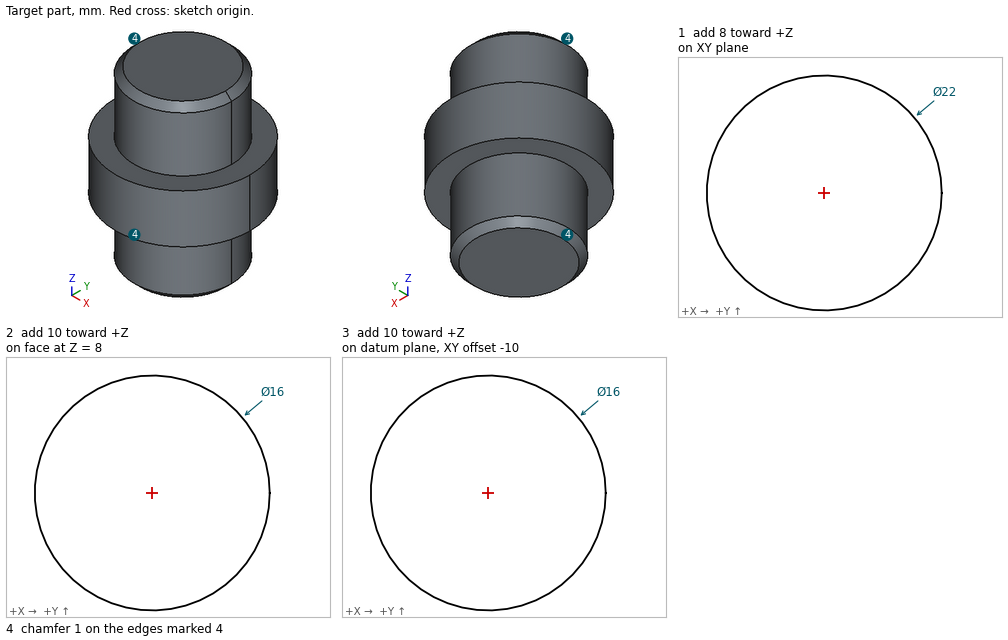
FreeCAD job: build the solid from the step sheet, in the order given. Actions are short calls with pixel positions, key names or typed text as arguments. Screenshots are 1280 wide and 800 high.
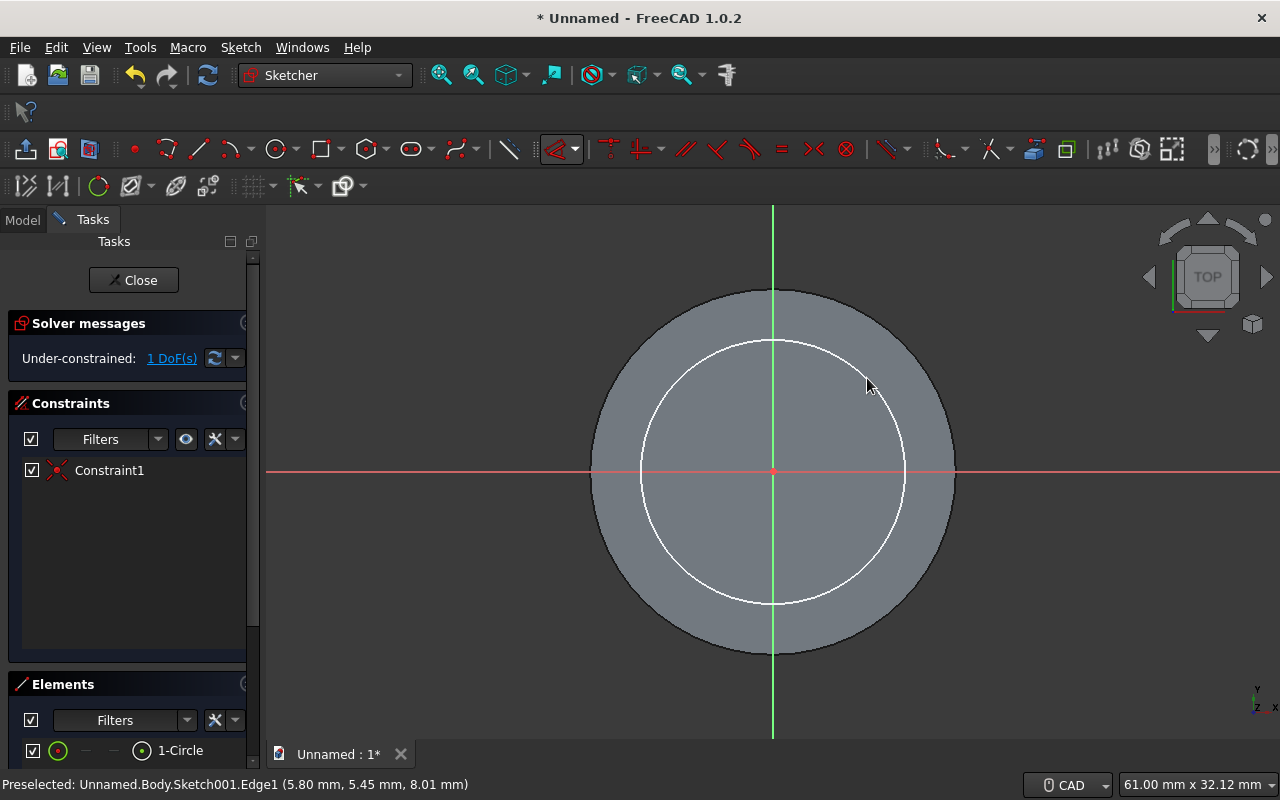
click(866, 378)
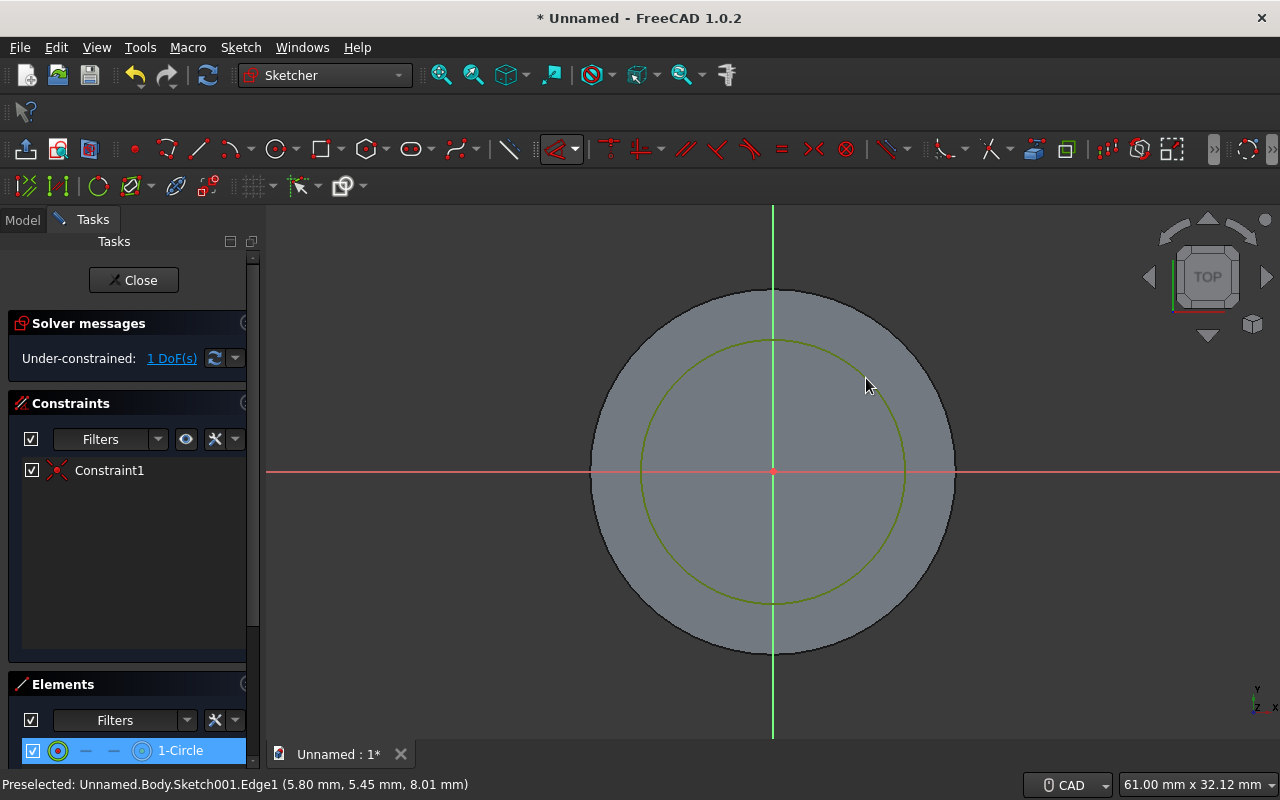
key(k)
key(o)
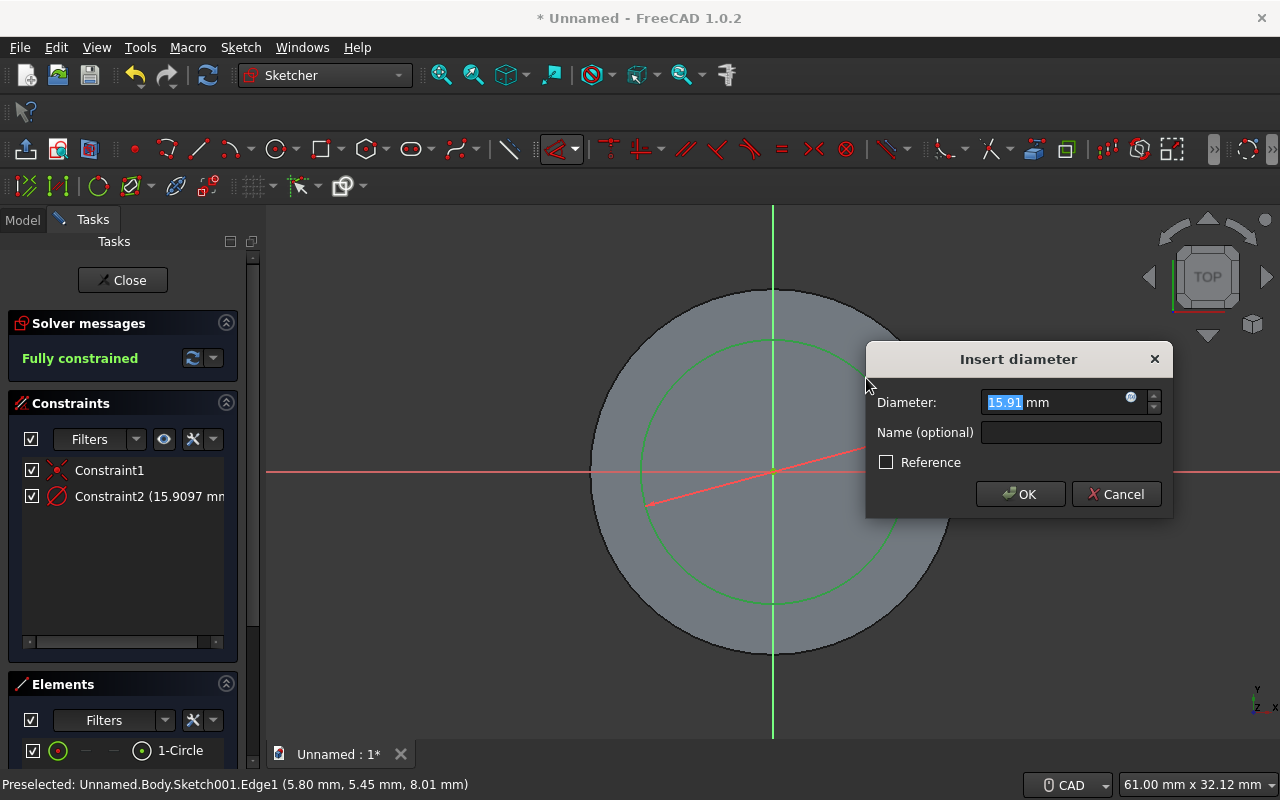
text(16)
key(Return)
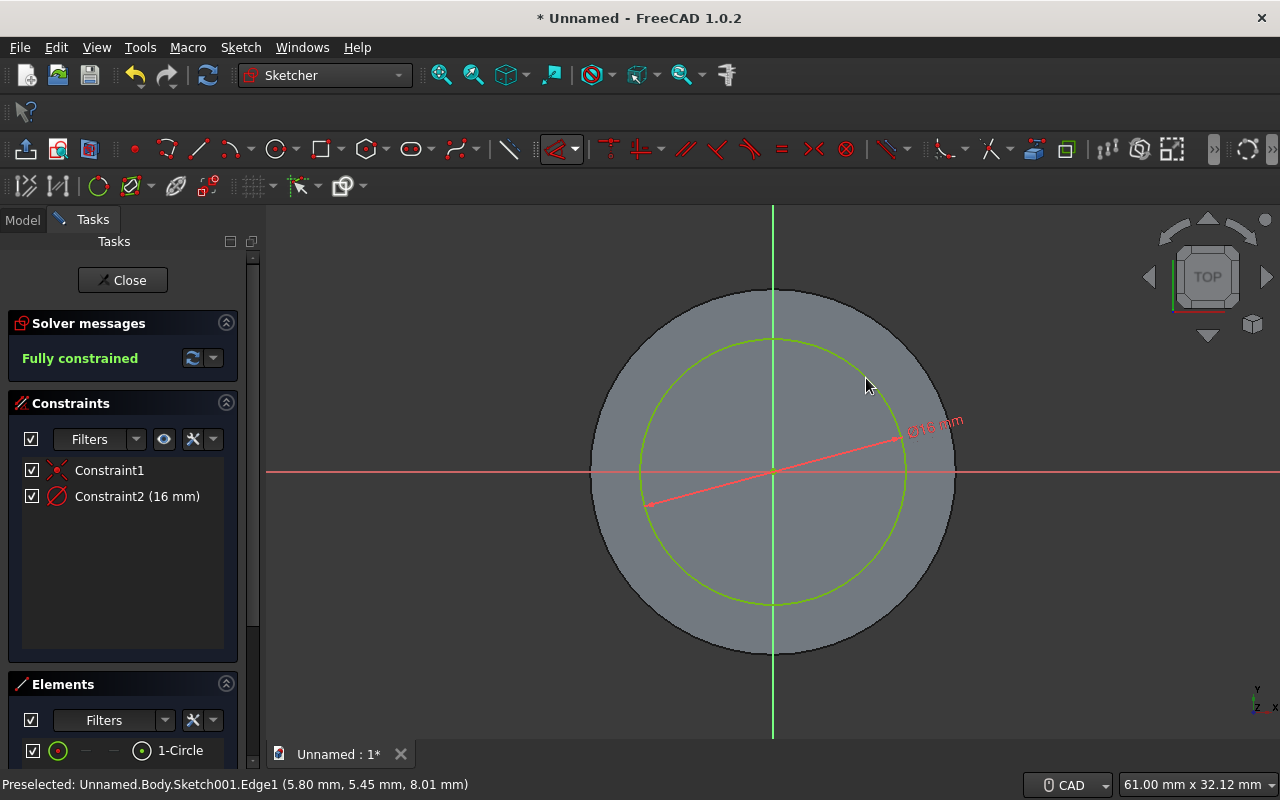
click(123, 280)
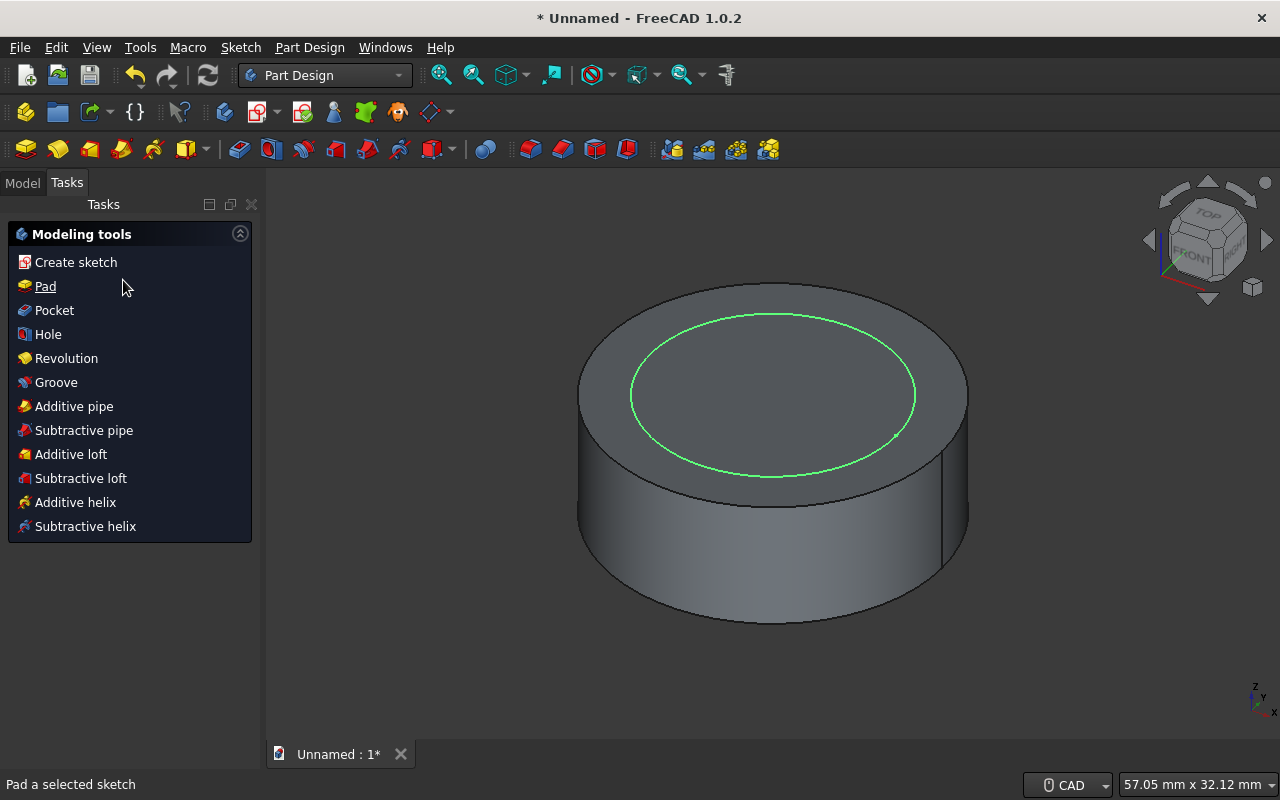
click(26, 150)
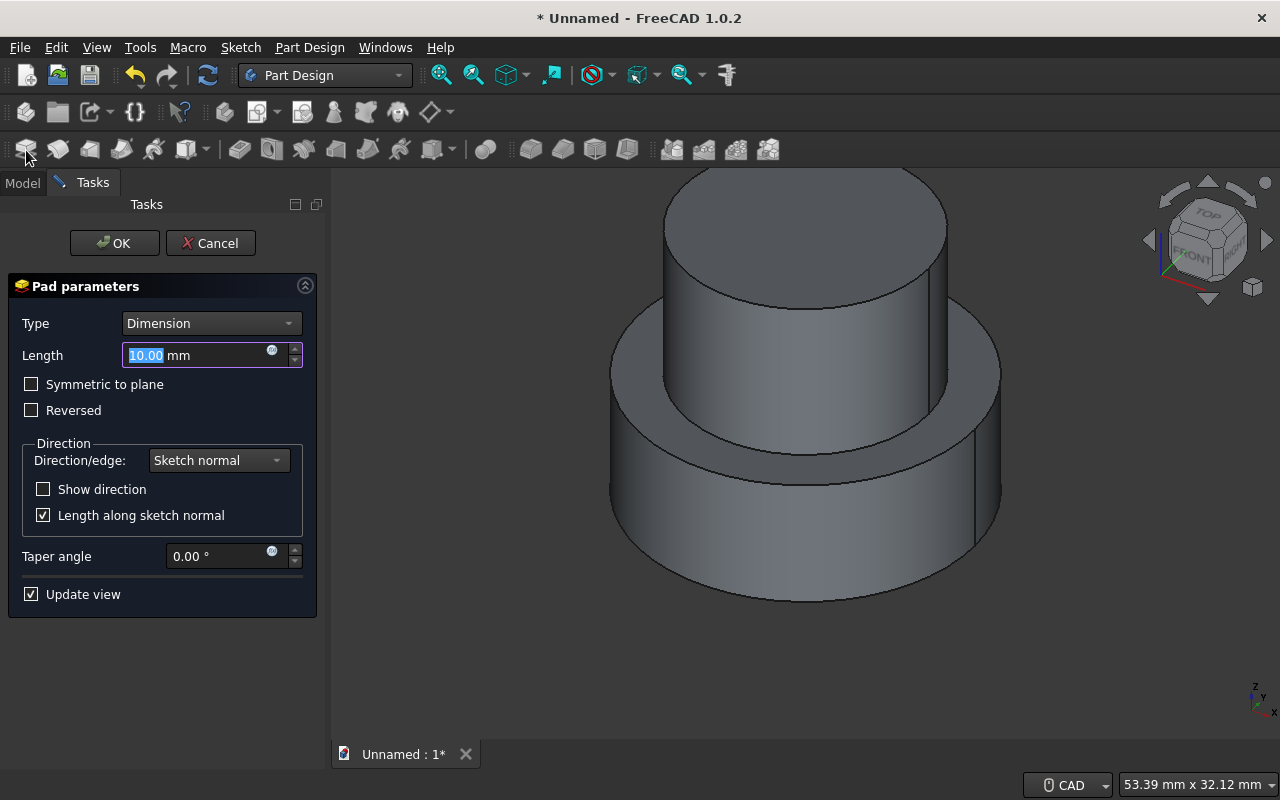
text(10)
key(Tab)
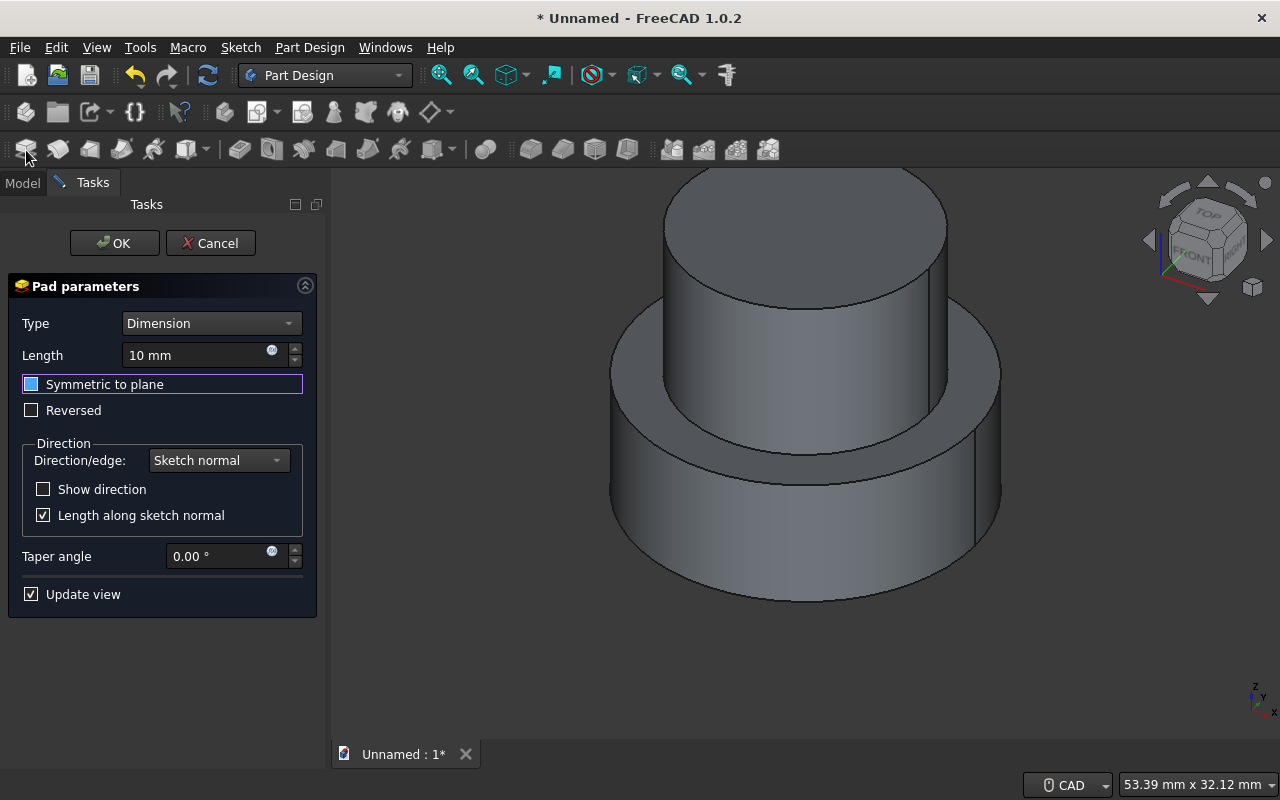
click(115, 243)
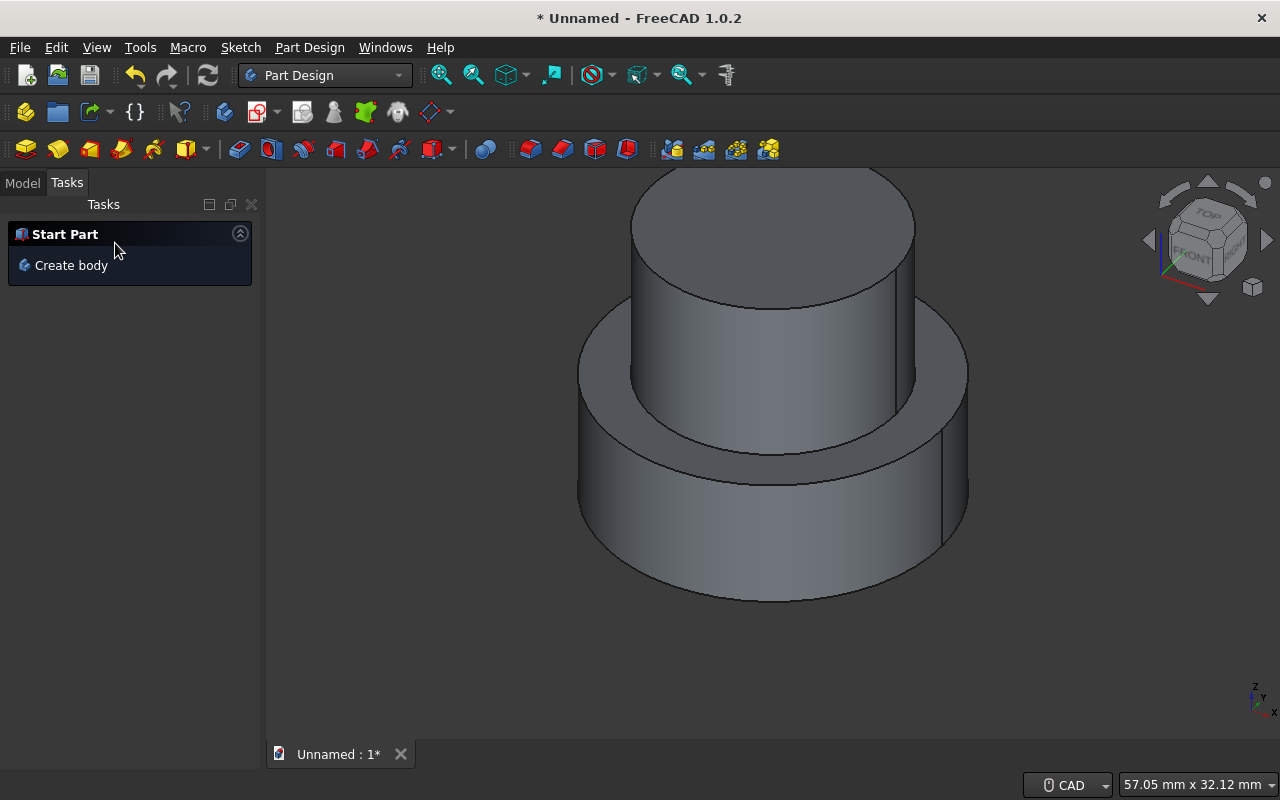
key(v)
key(f)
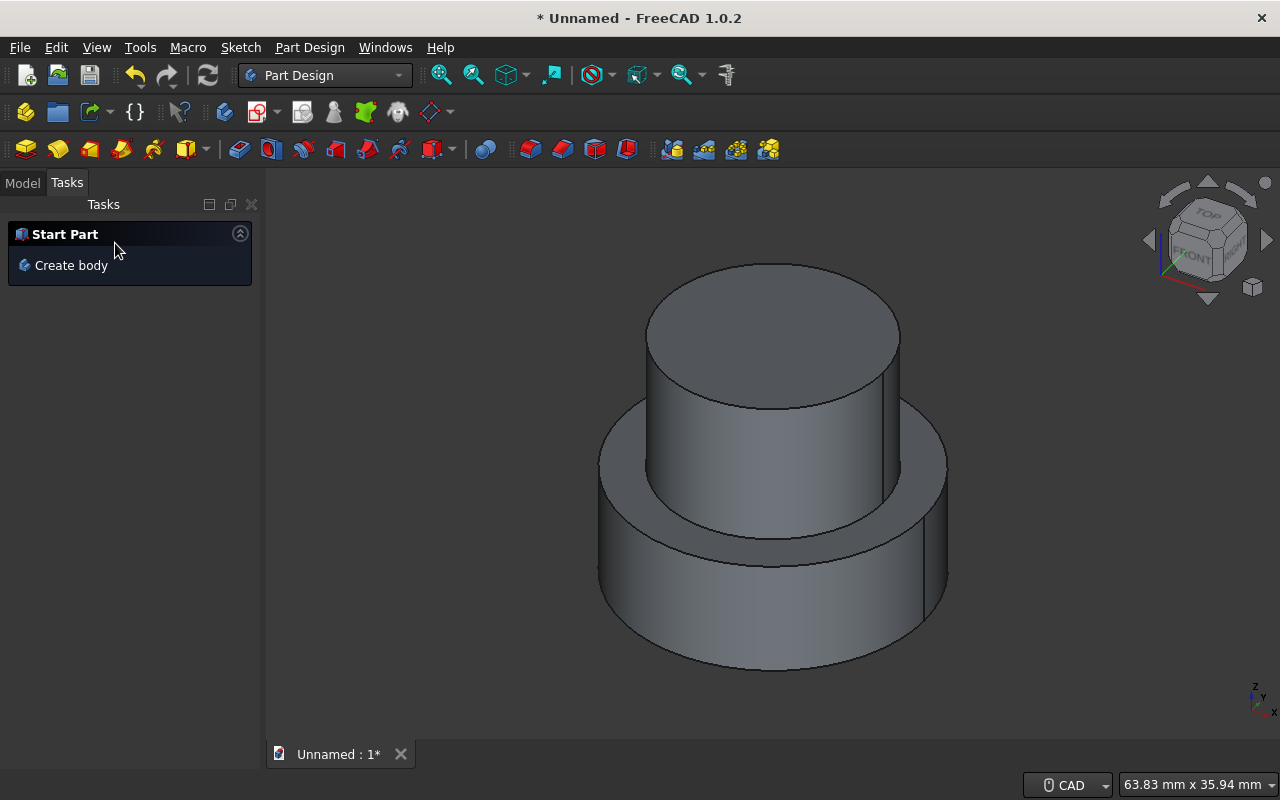
click(23, 182)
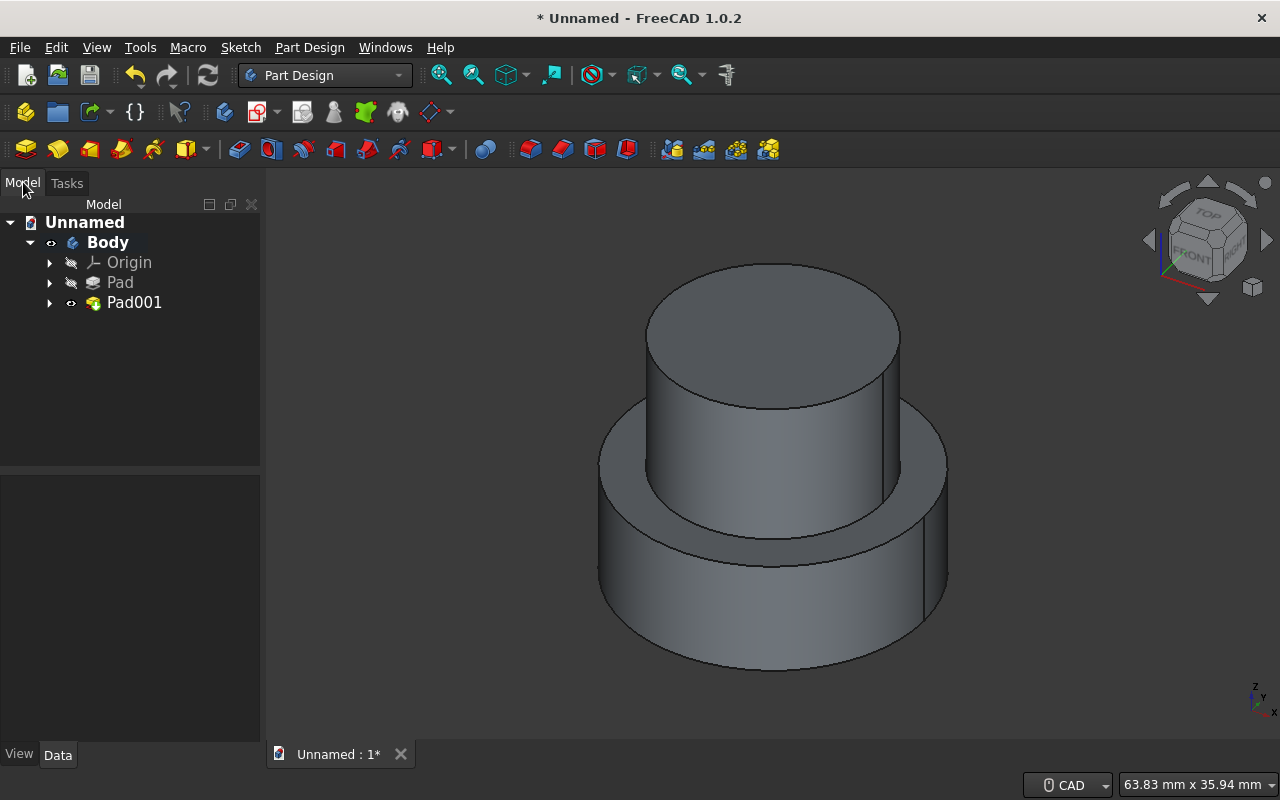
click(50, 263)